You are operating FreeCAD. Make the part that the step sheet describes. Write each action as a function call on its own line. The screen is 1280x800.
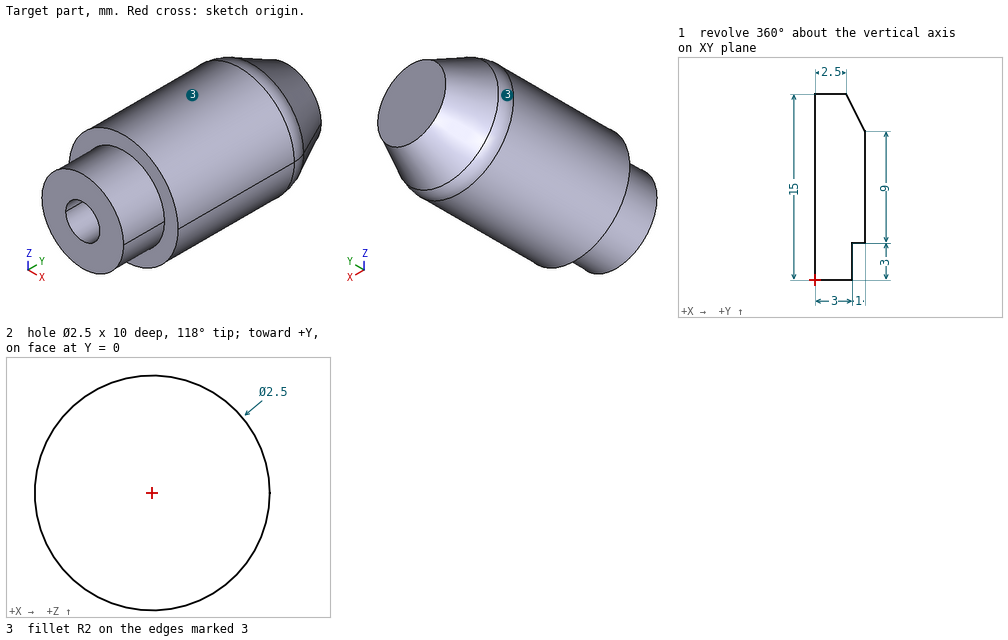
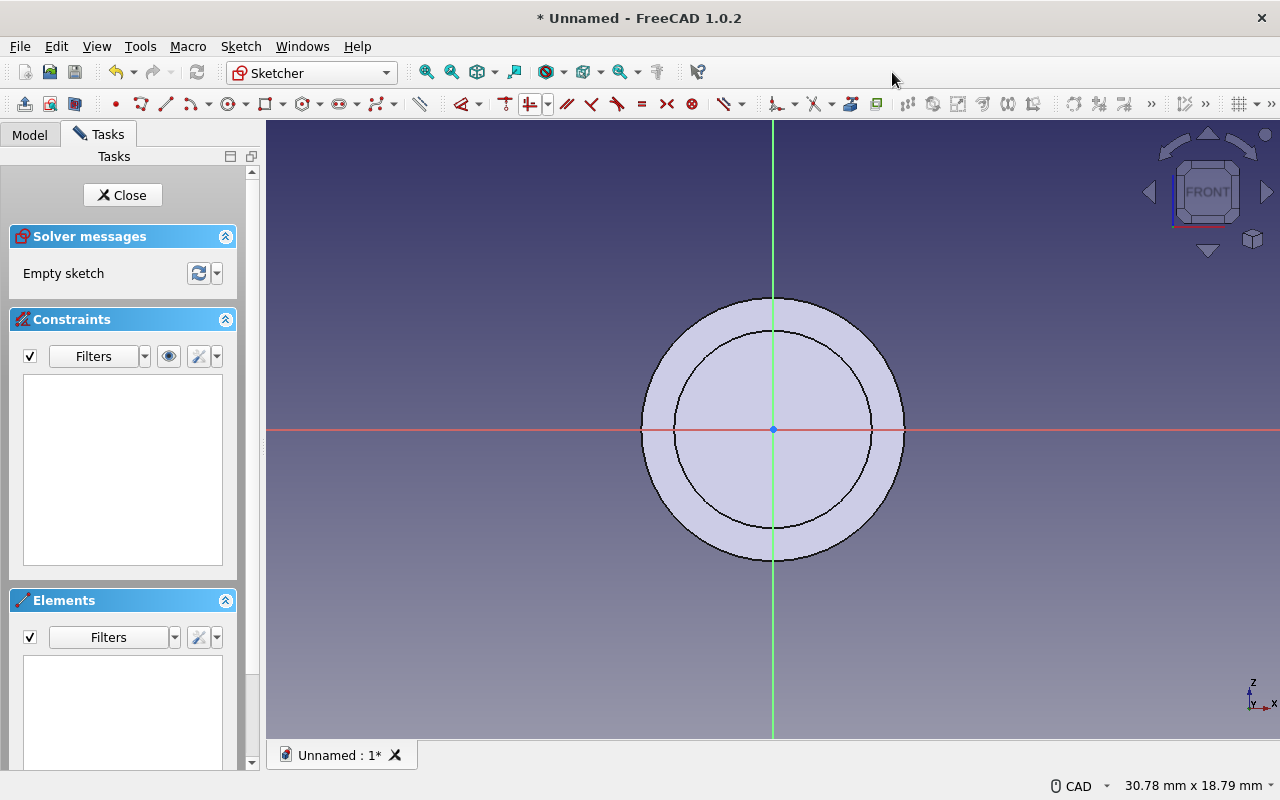
scroll(790, 430, up, 8)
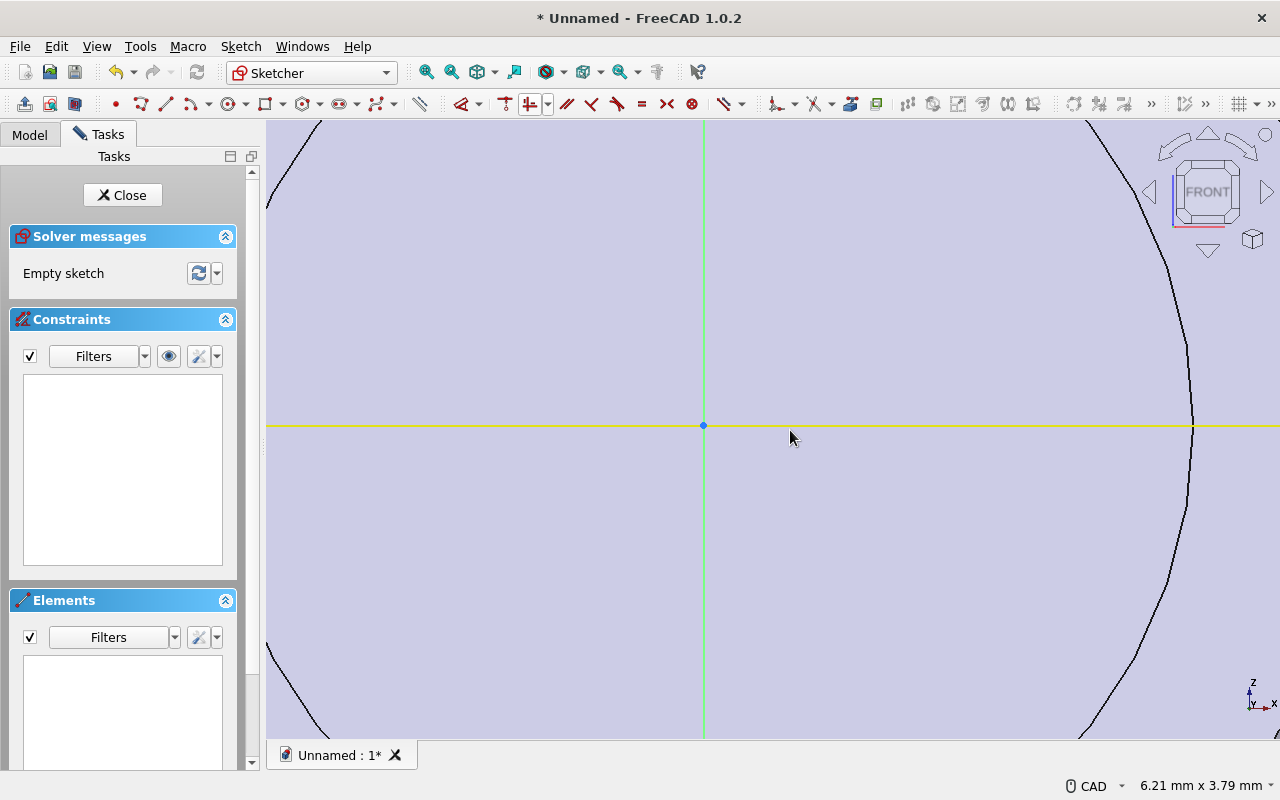
click(228, 104)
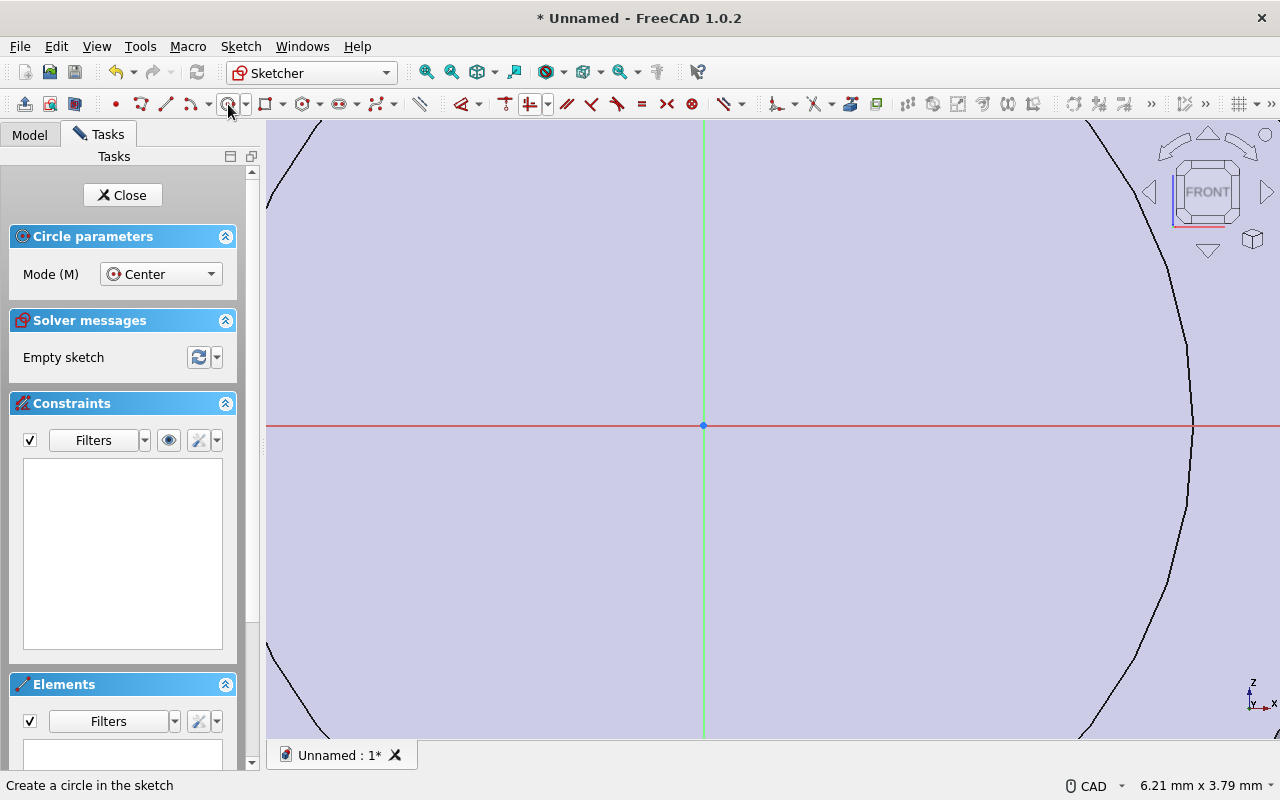
click(704, 426)
move(848, 281)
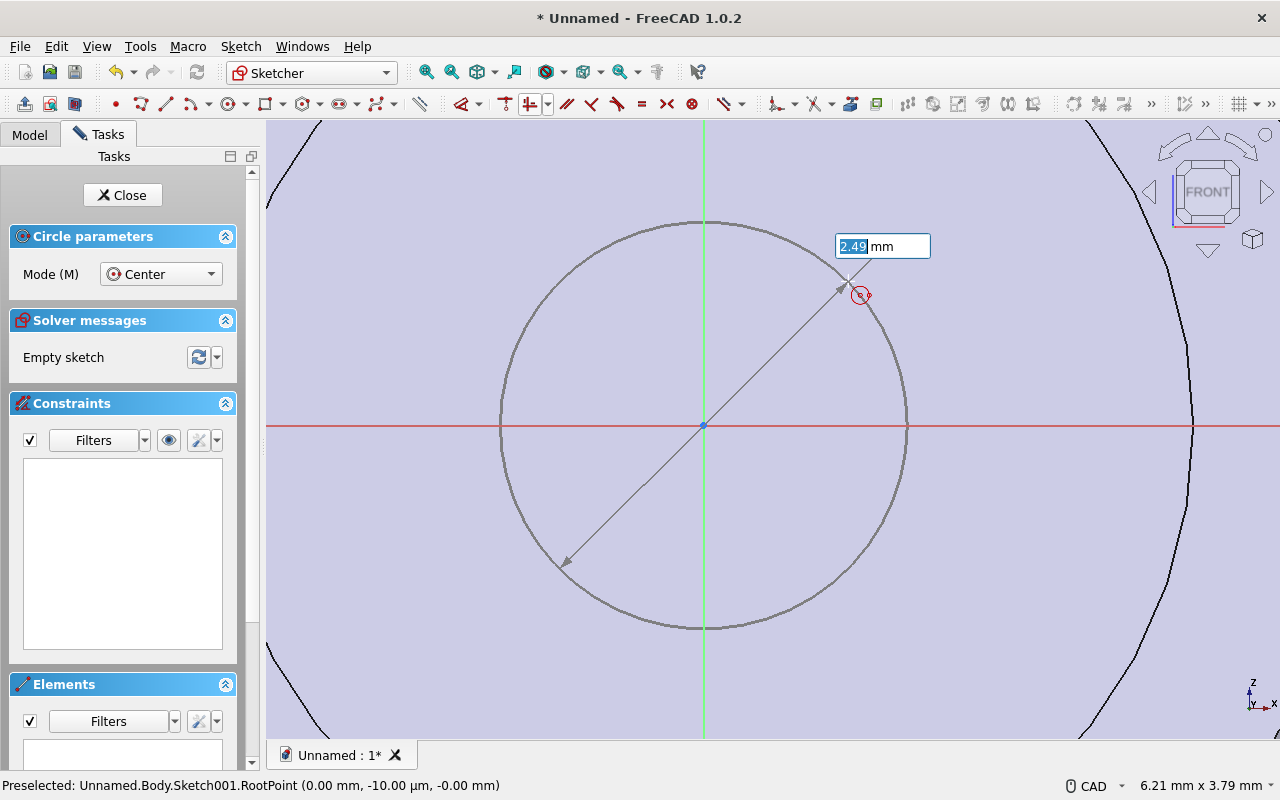
text(2.5)
key(Return)
key(Escape)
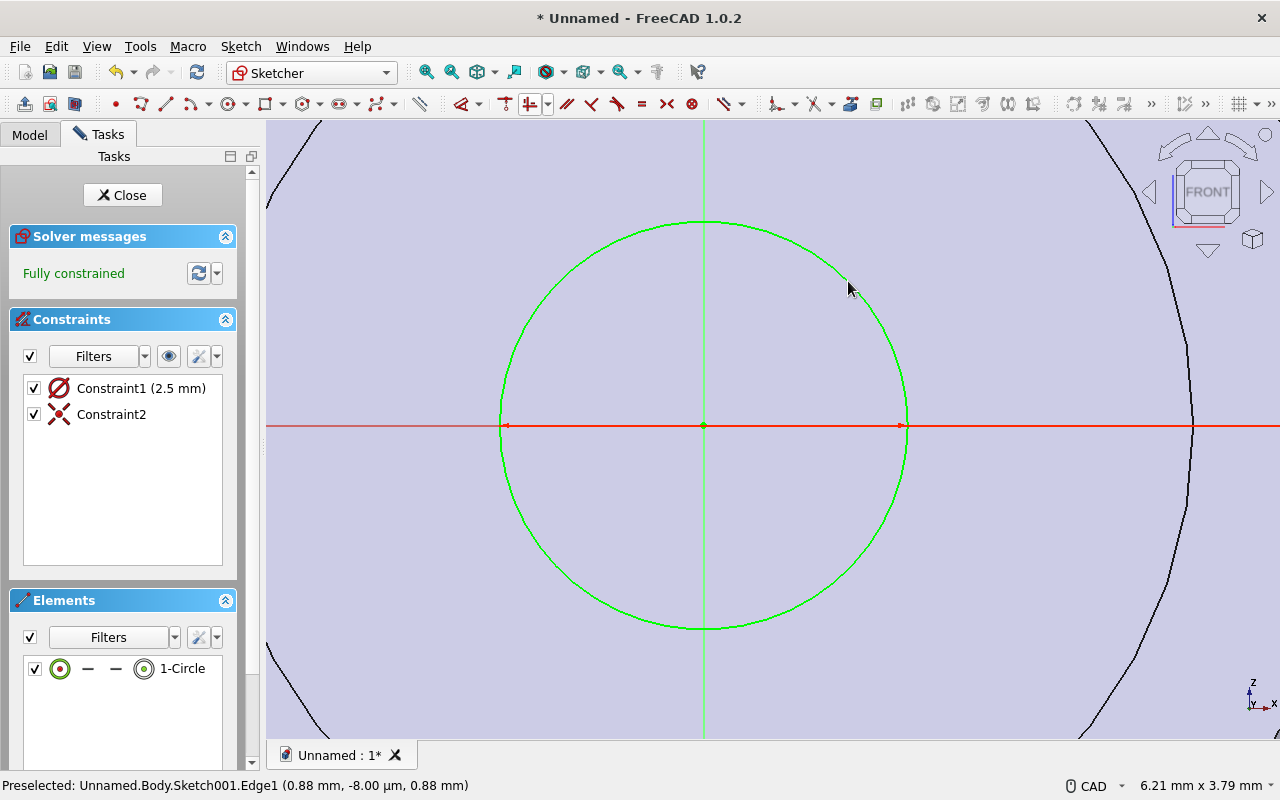
click(123, 195)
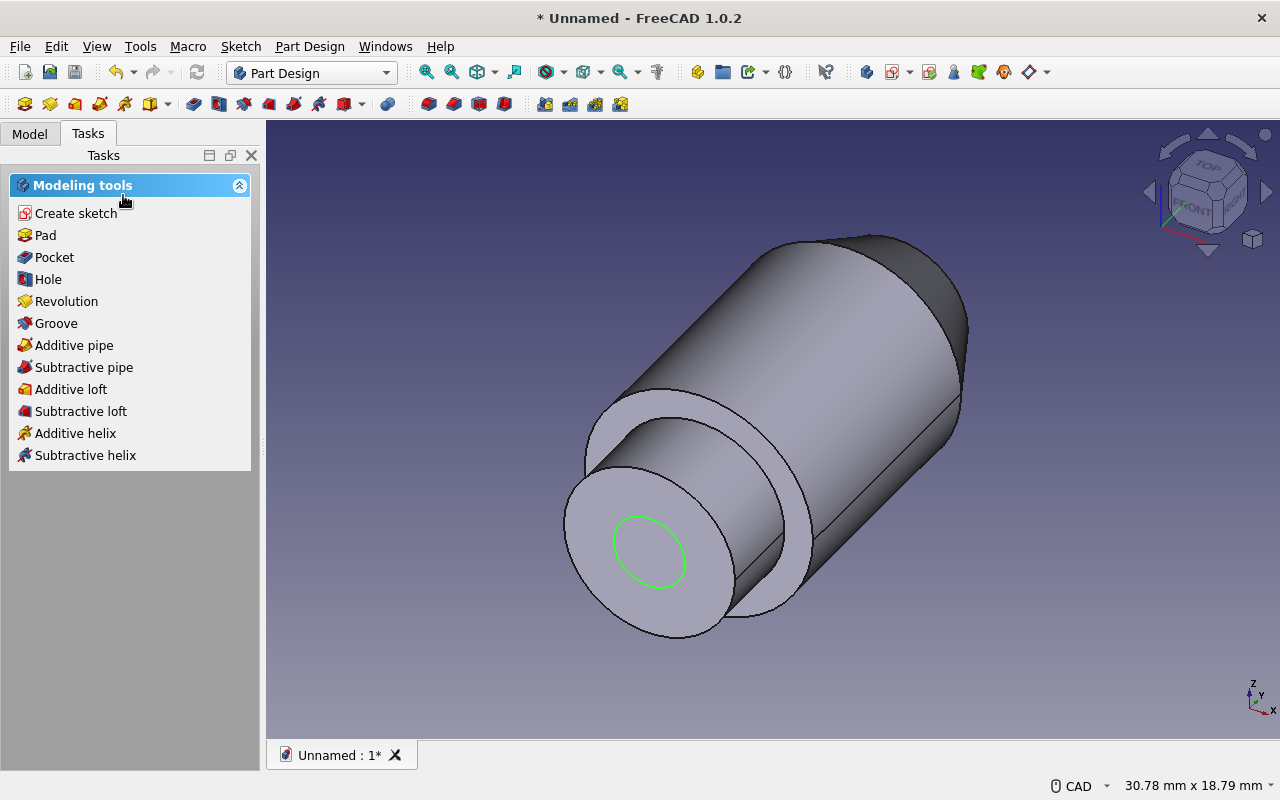
click(219, 104)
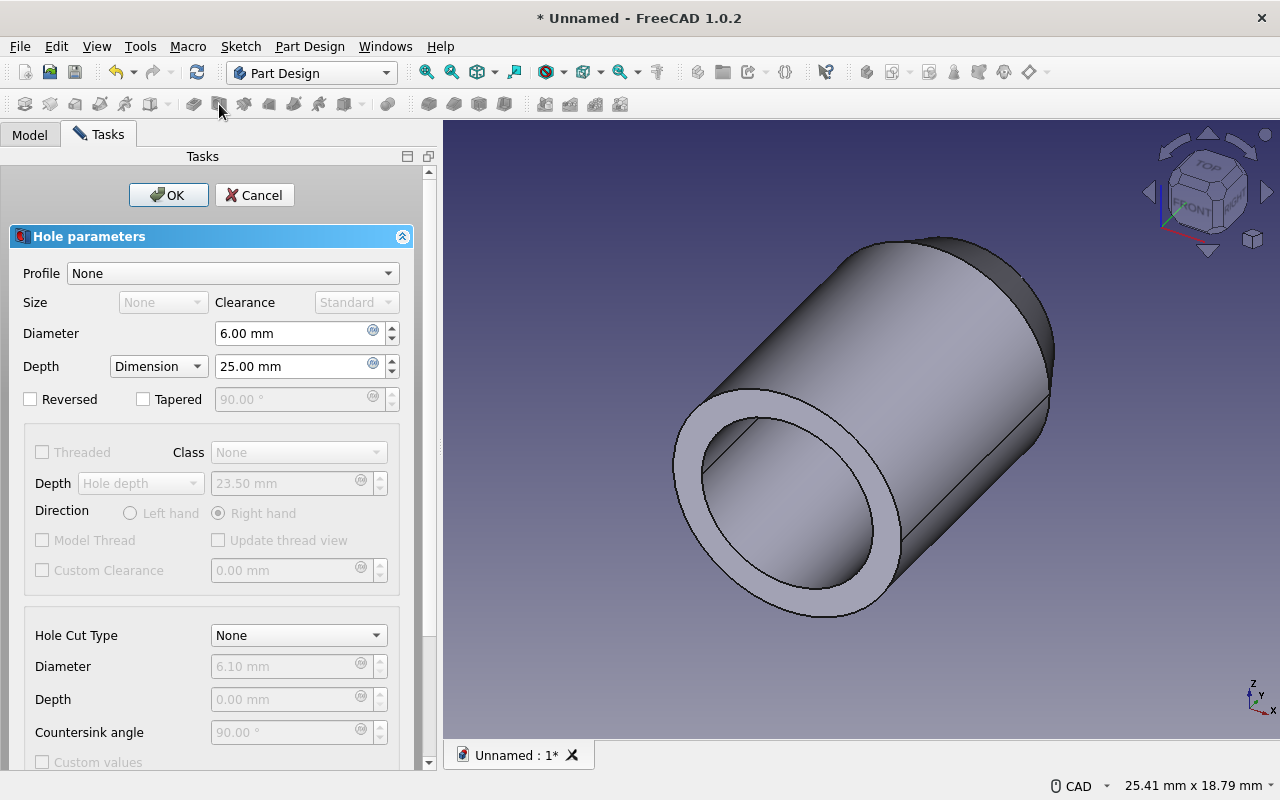
triple_click(300, 334)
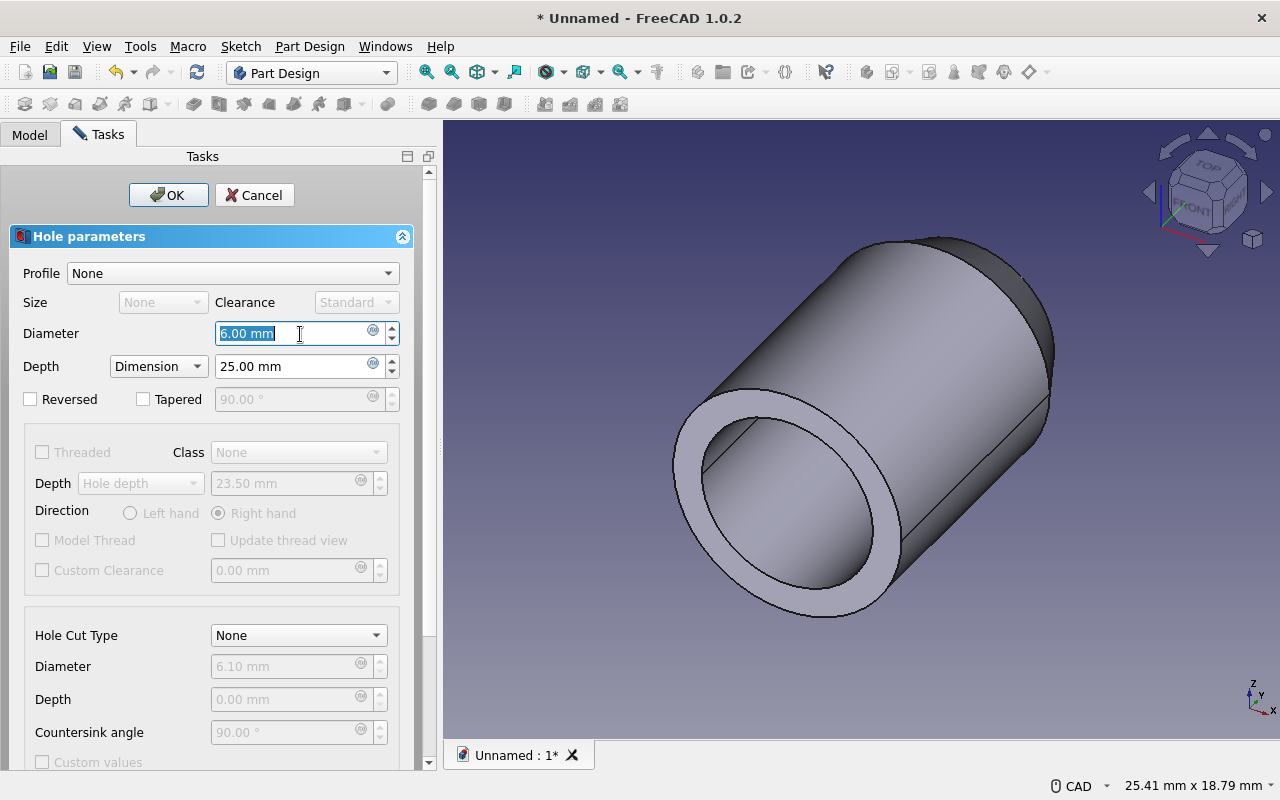
text(2.5)
key(Tab)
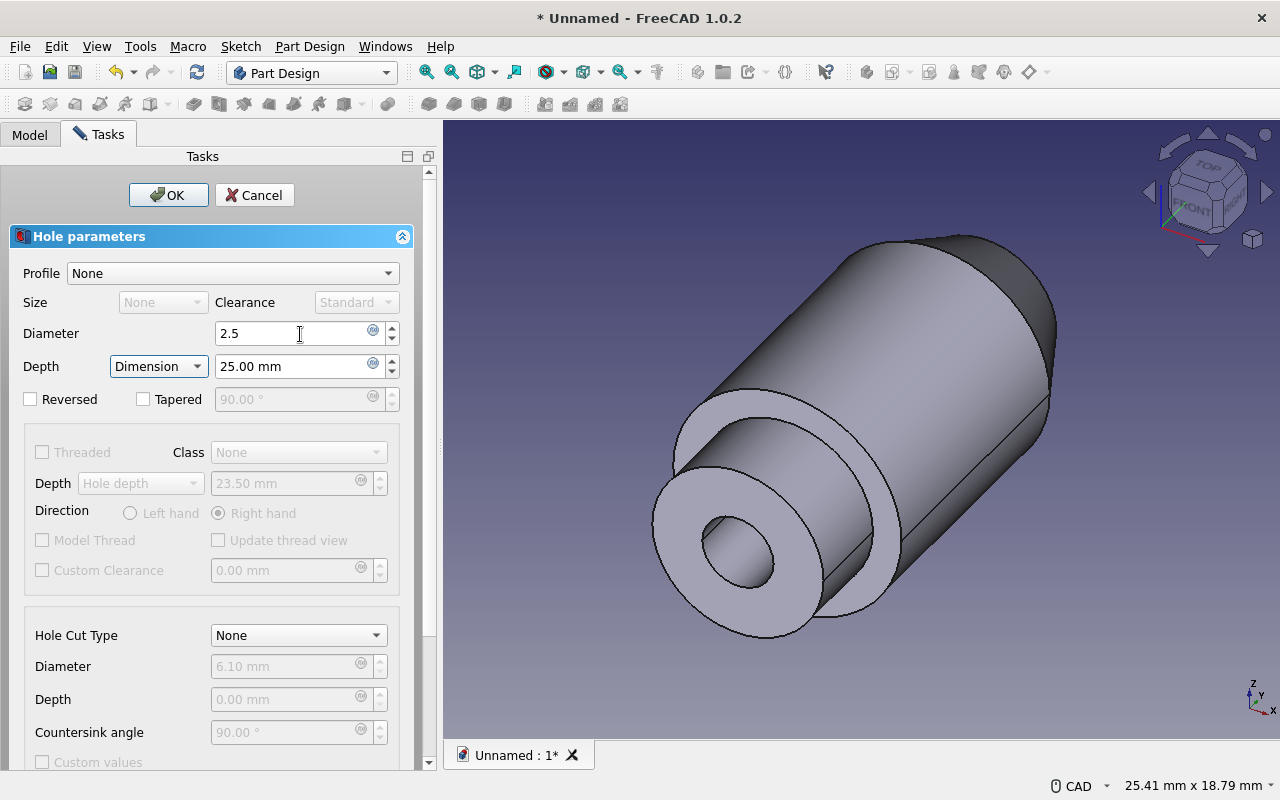
triple_click(300, 366)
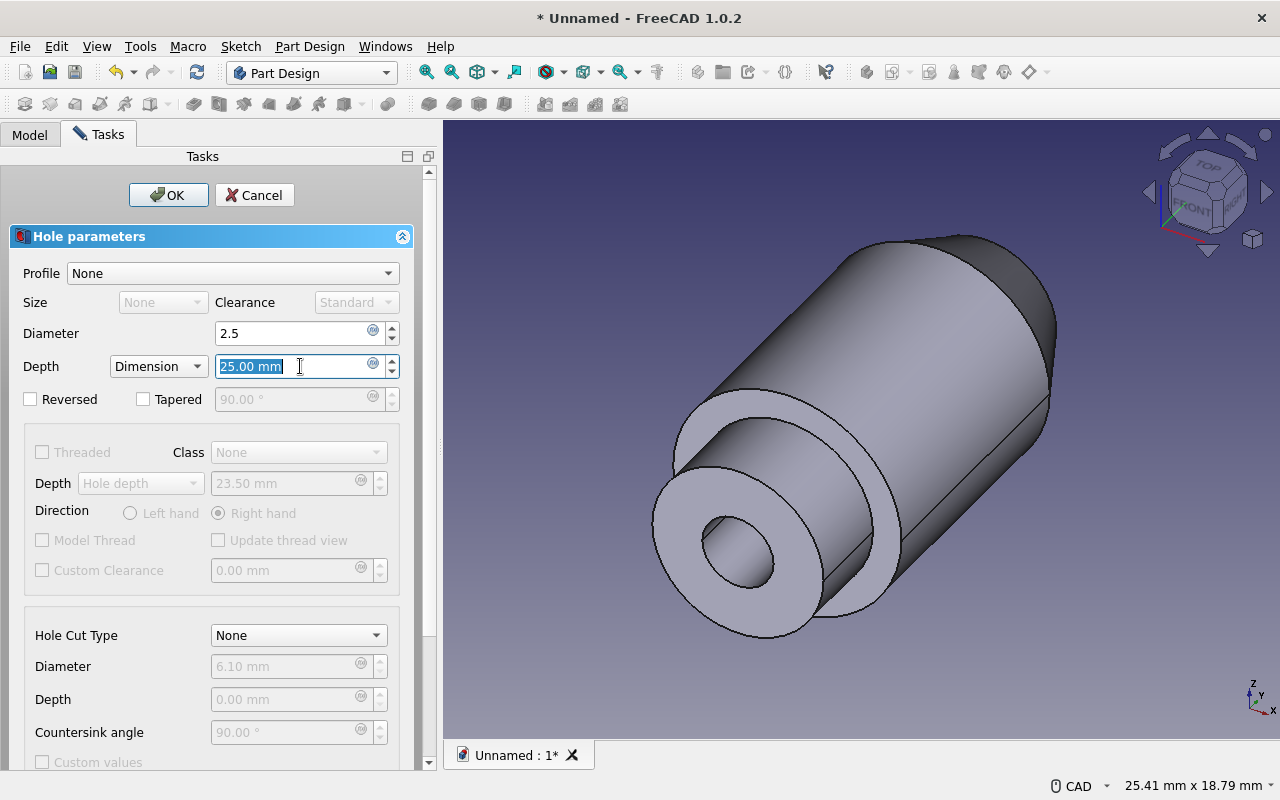
text(10)
key(Tab)